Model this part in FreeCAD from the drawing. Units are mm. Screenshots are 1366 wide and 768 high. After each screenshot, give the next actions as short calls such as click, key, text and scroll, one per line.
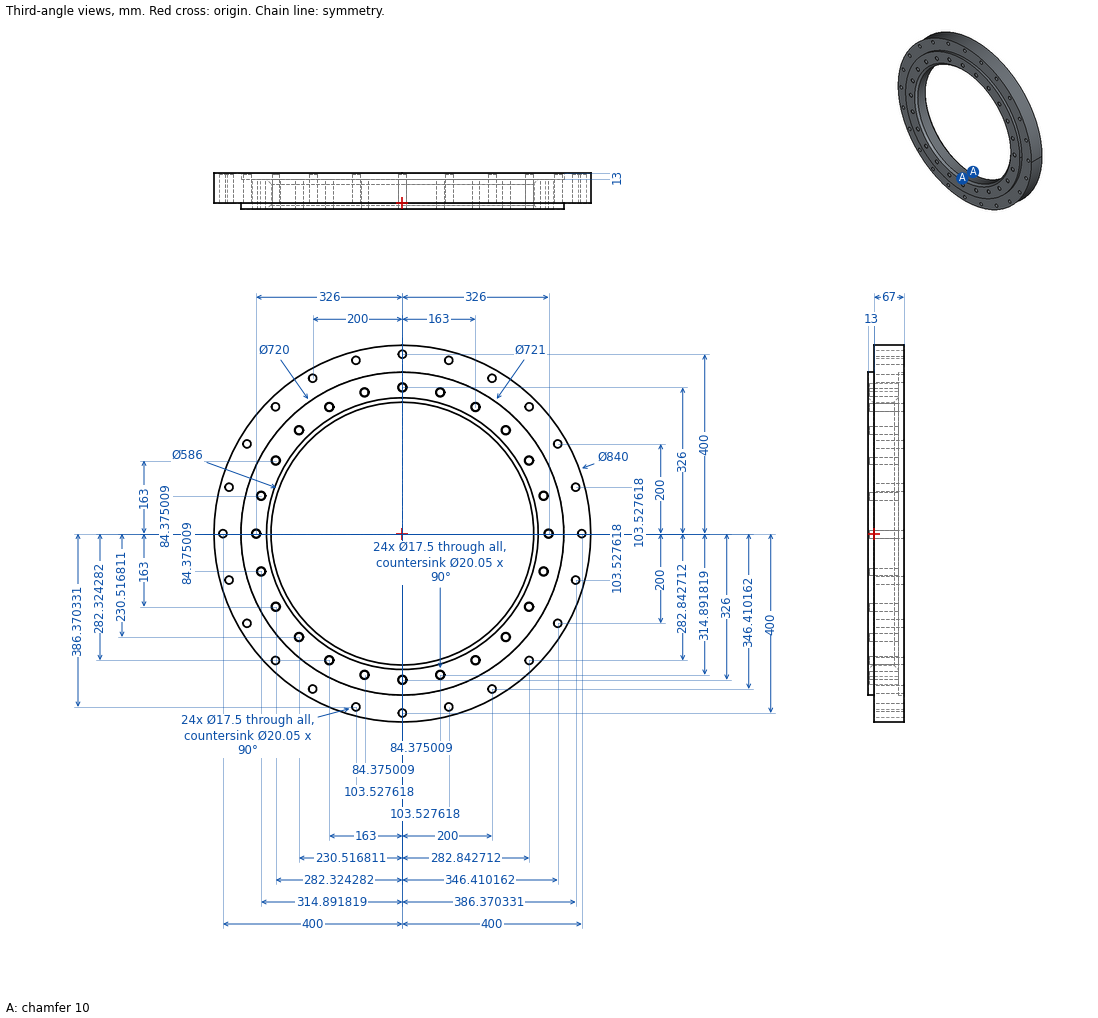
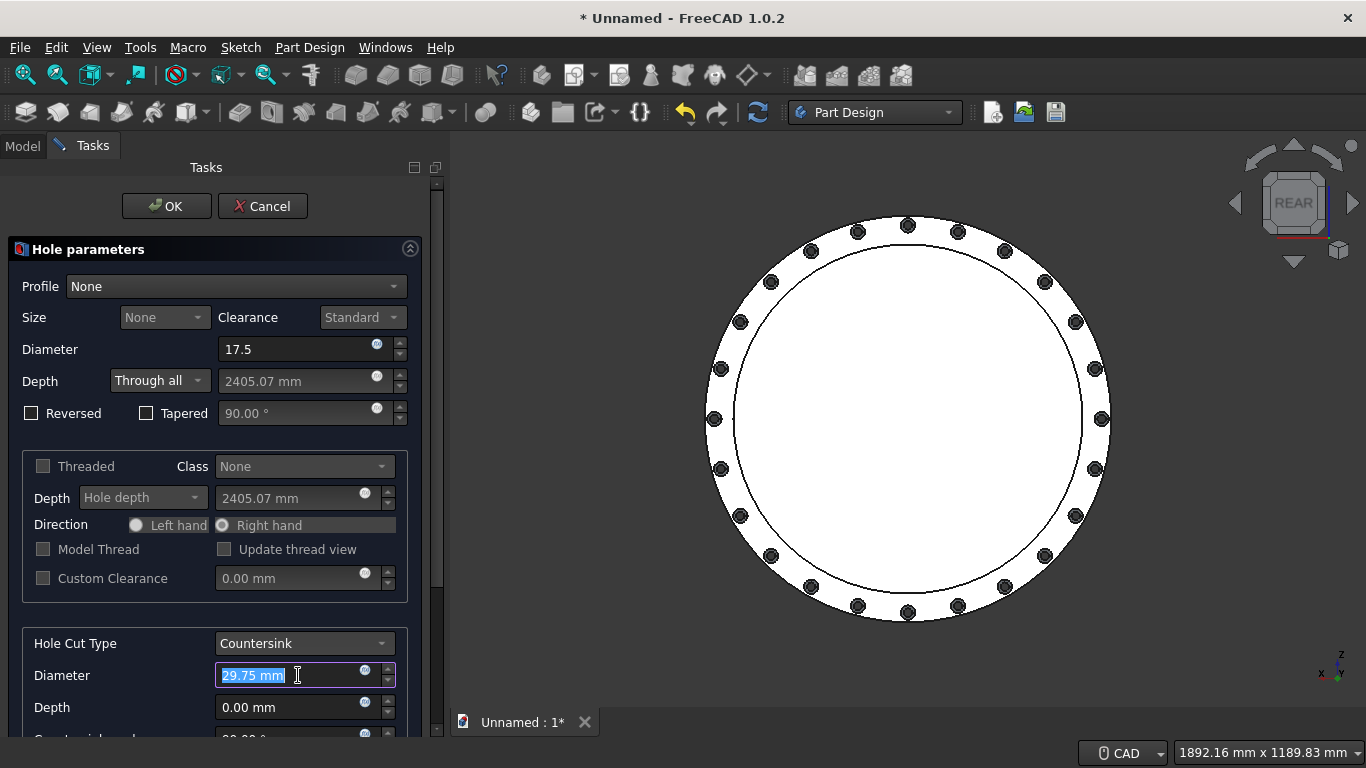
text(20.05)
key(Tab)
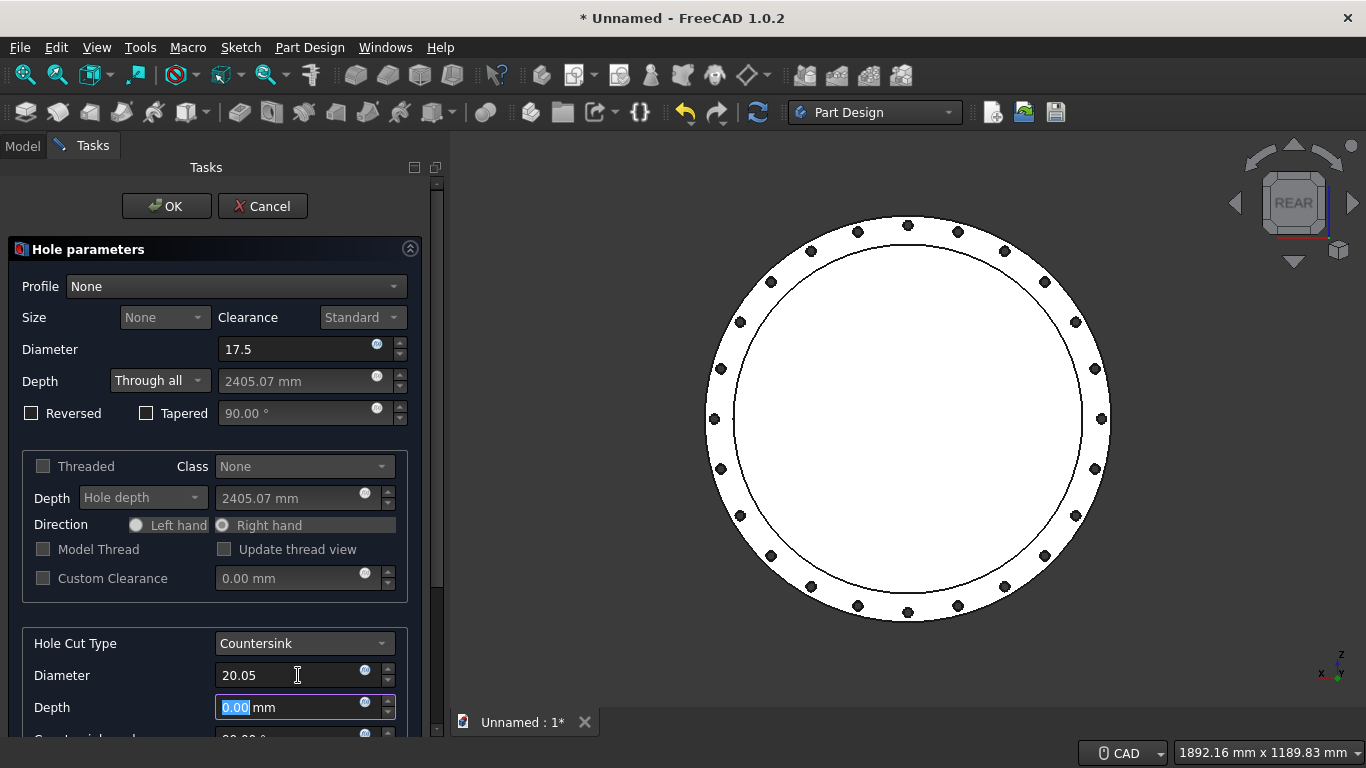
click(167, 206)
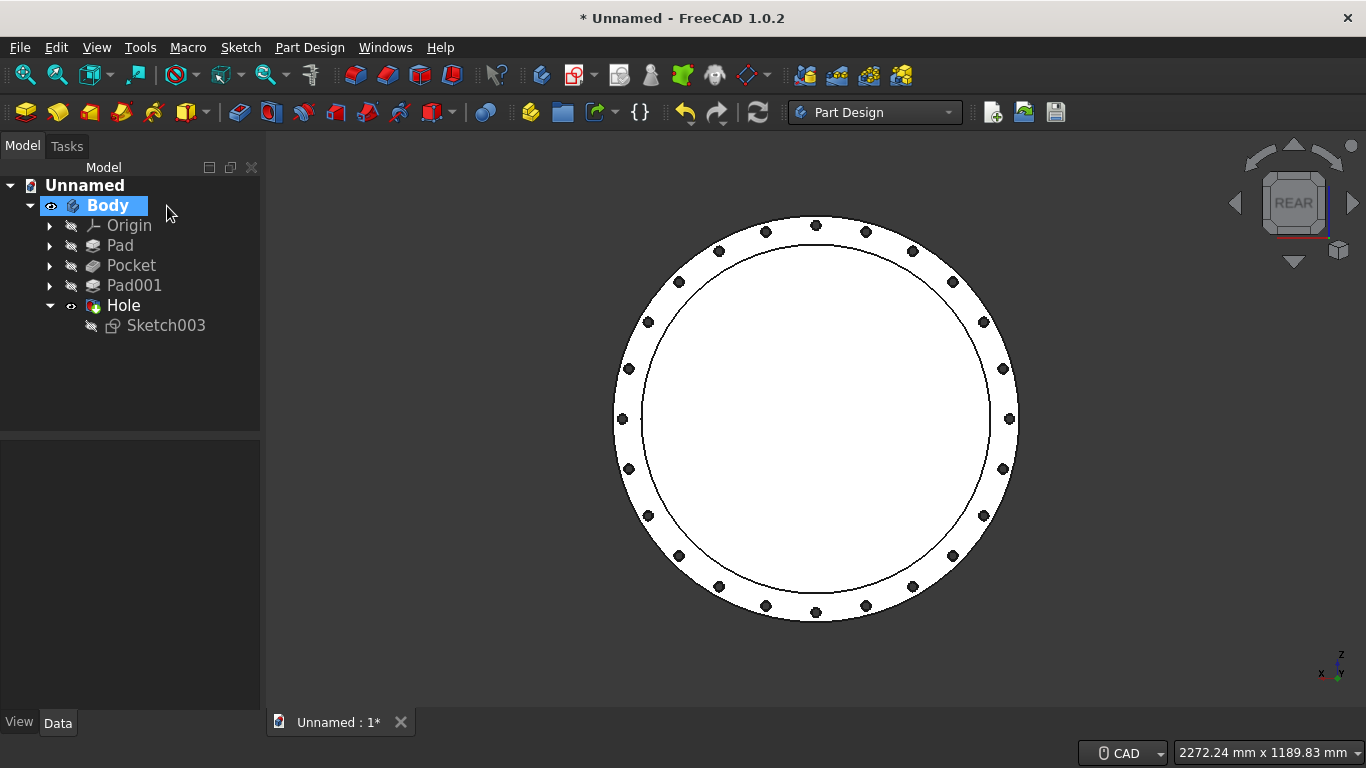
click(816, 418)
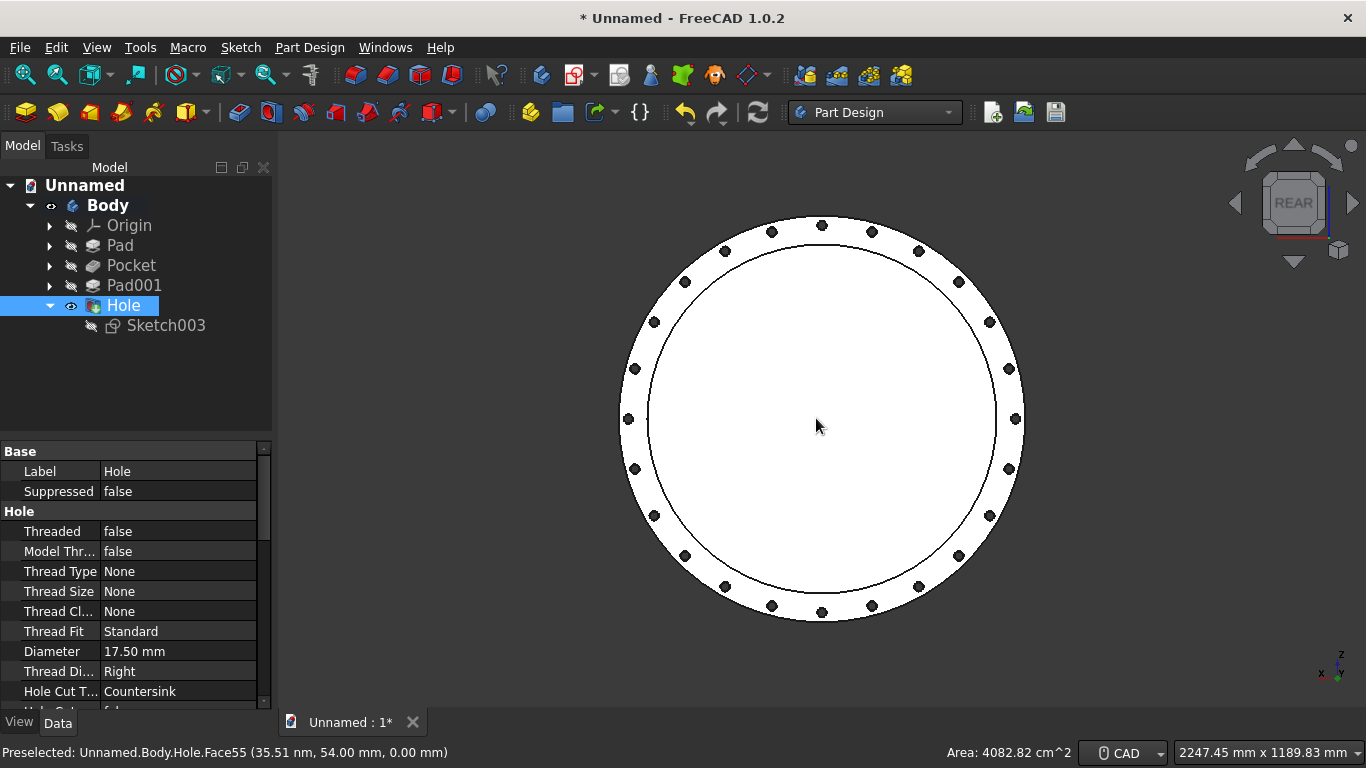
click(574, 76)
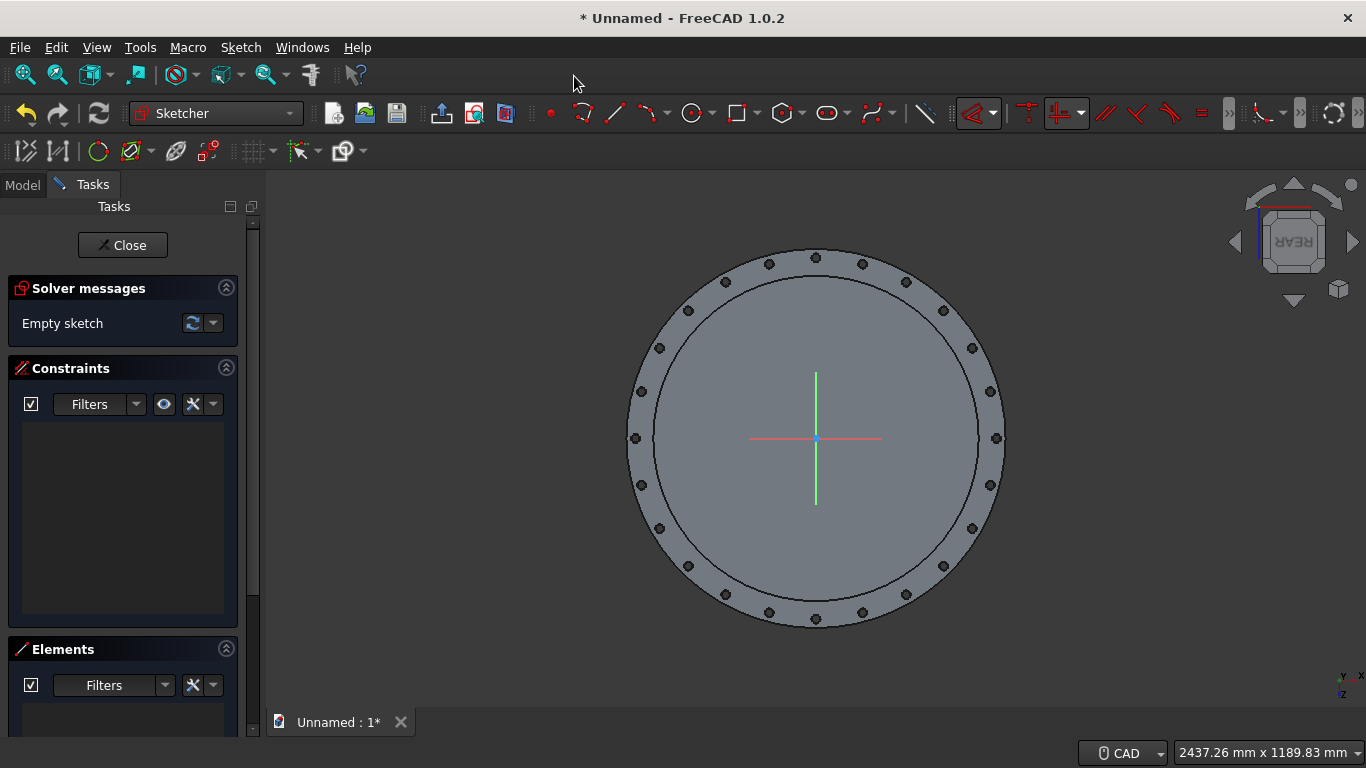
click(506, 114)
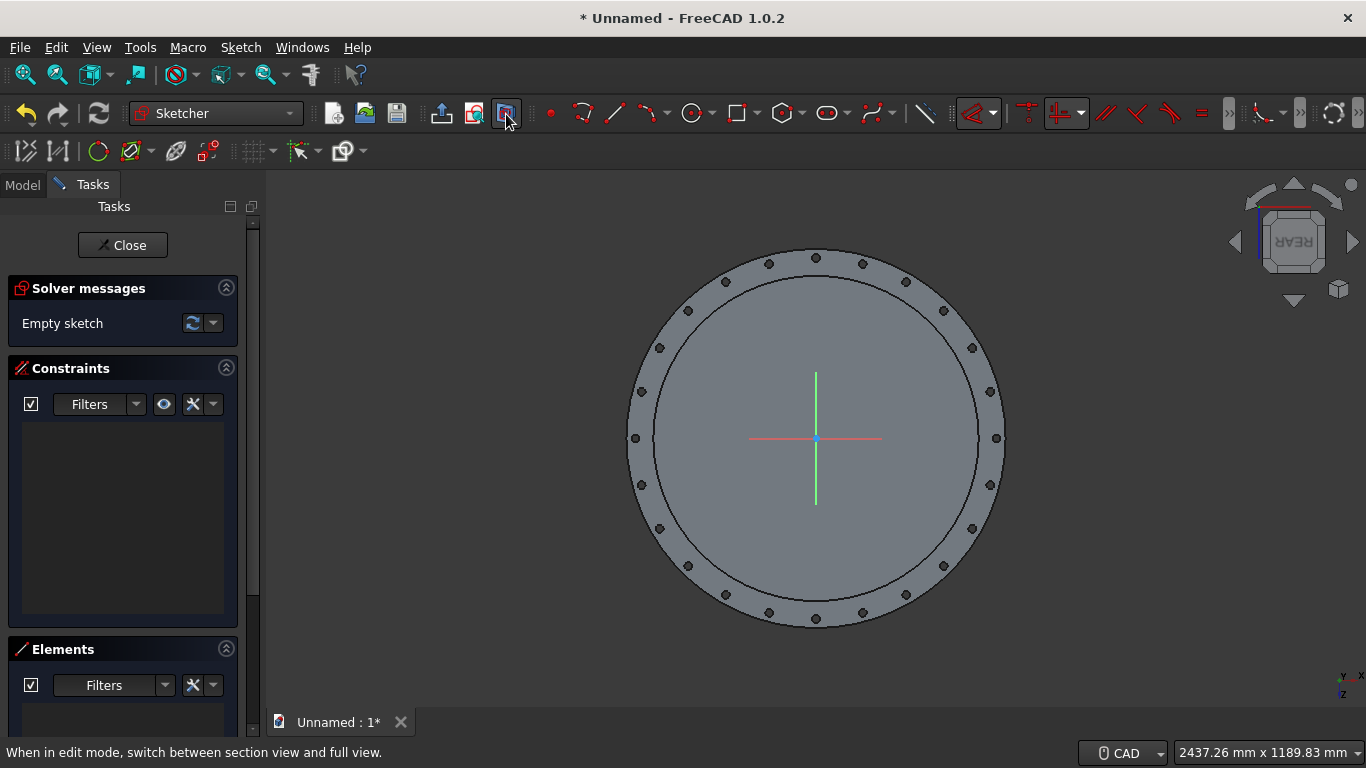
click(692, 114)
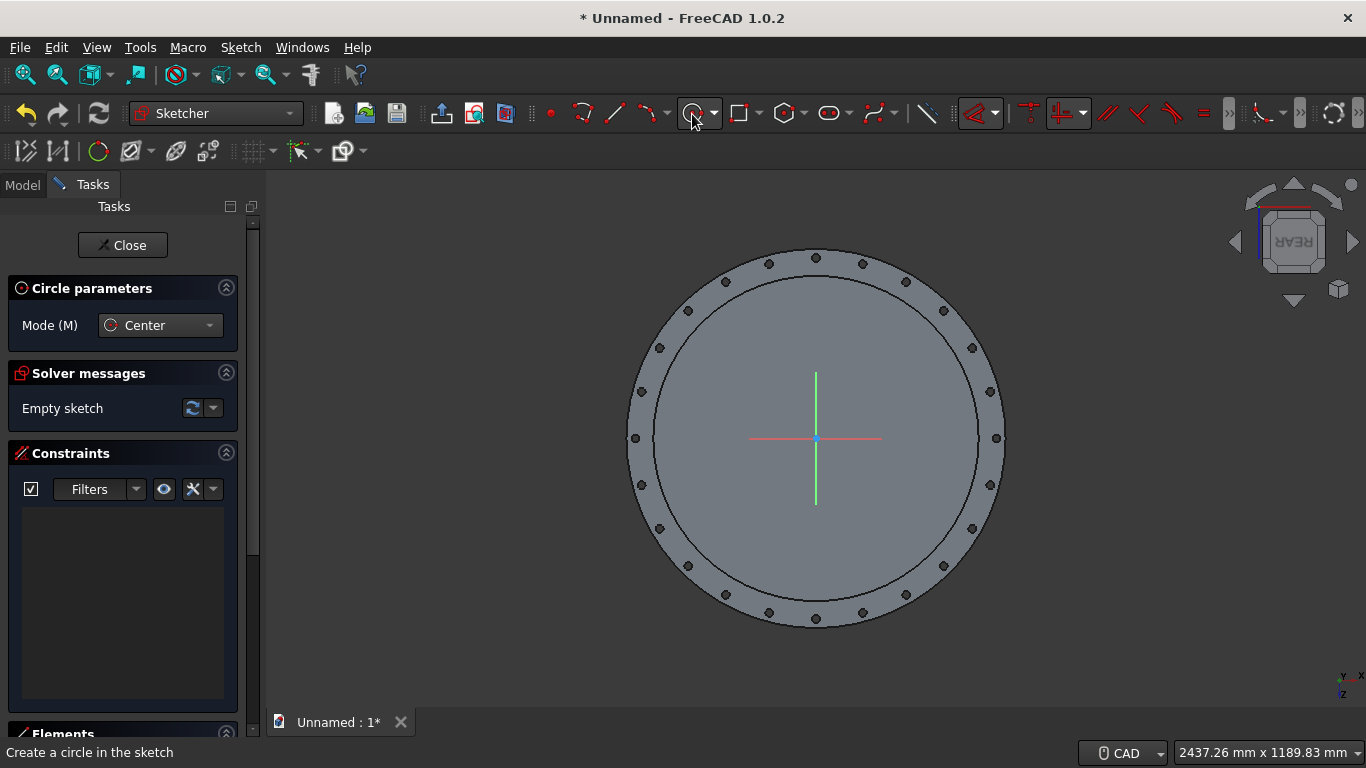
click(816, 438)
click(910, 345)
key(Escape)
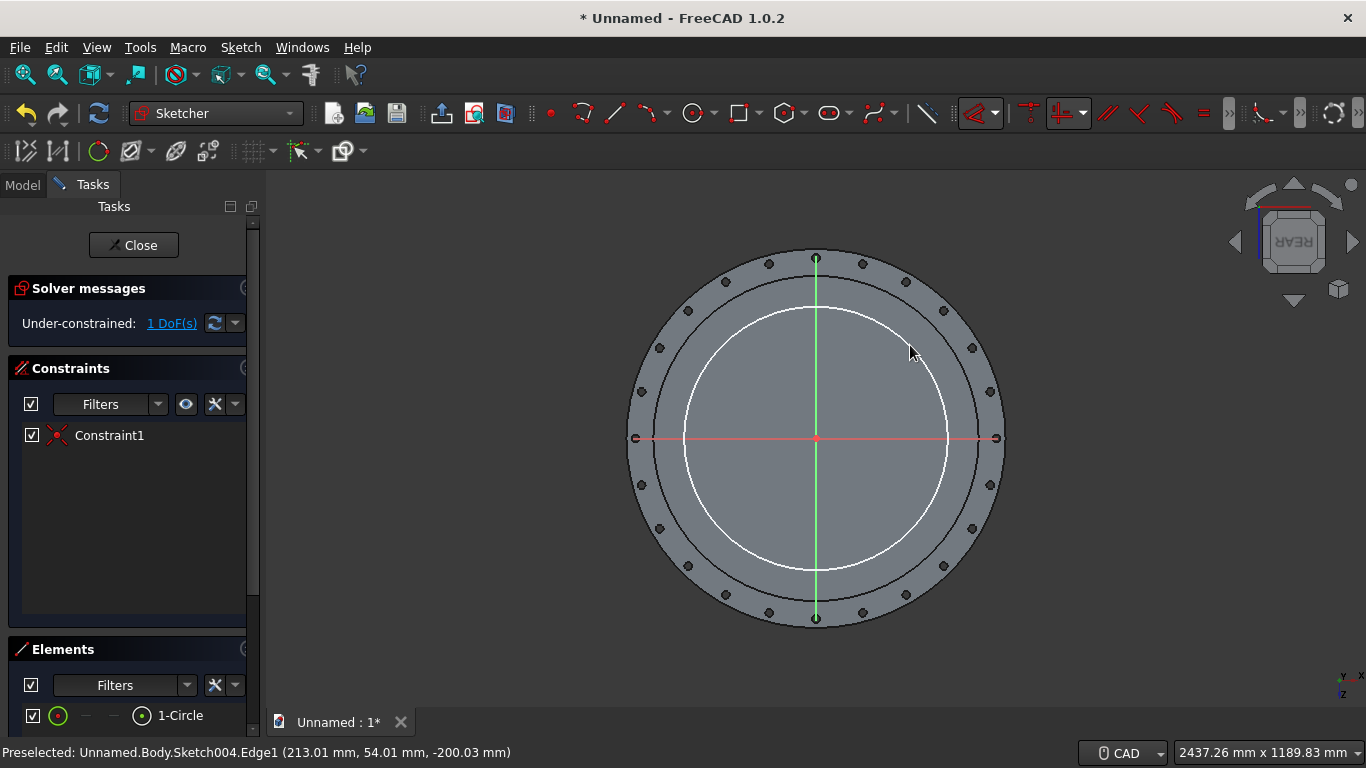
click(909, 345)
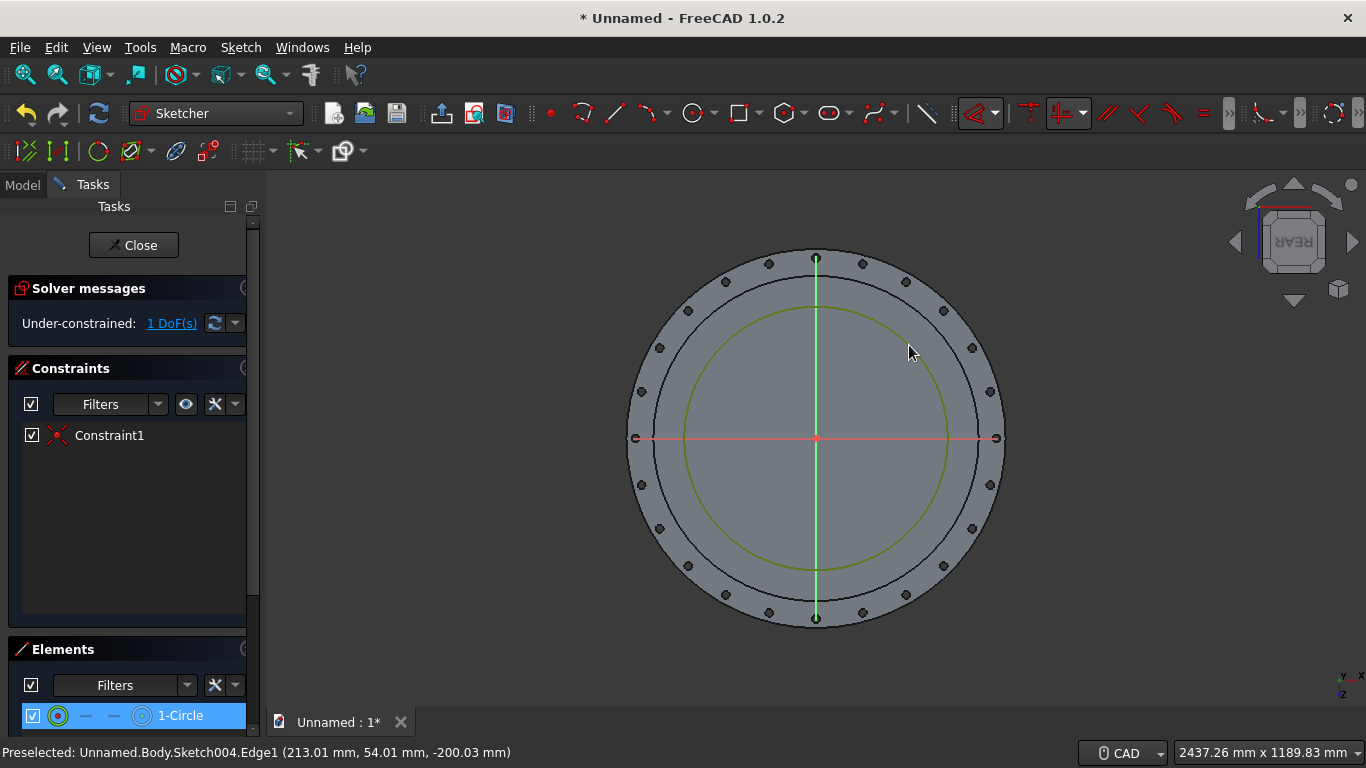
click(998, 114)